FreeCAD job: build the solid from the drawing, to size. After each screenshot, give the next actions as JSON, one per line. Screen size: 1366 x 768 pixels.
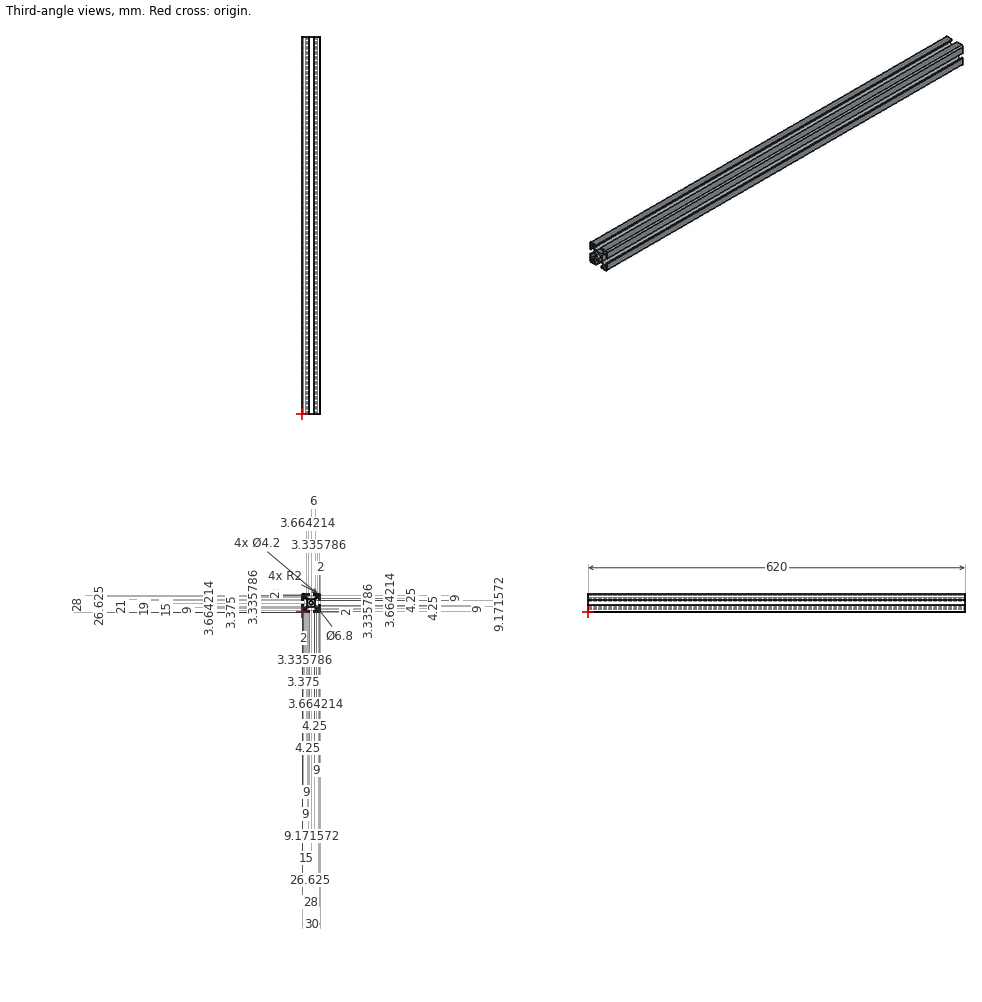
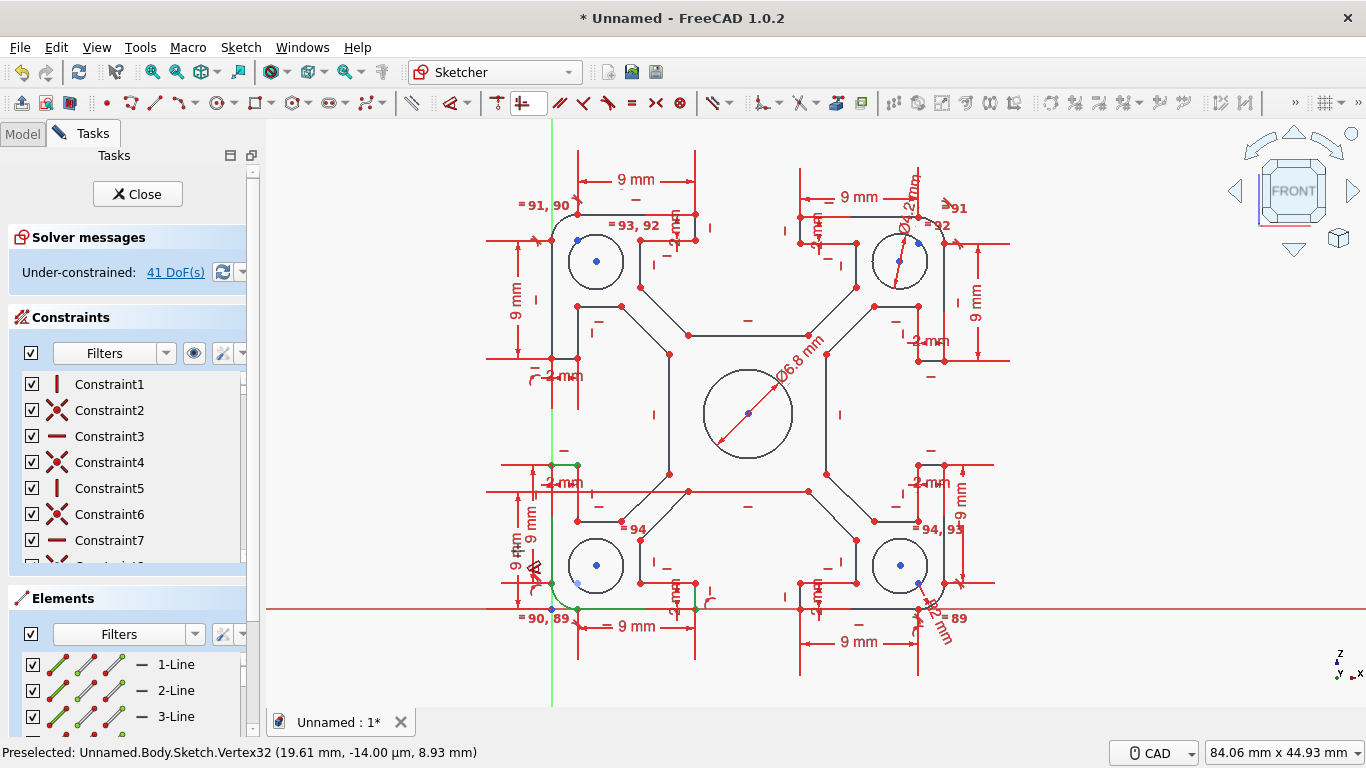
{"action": "left_click", "coordinate": [669, 475]}
{"action": "left_click", "coordinate": [610, 441]}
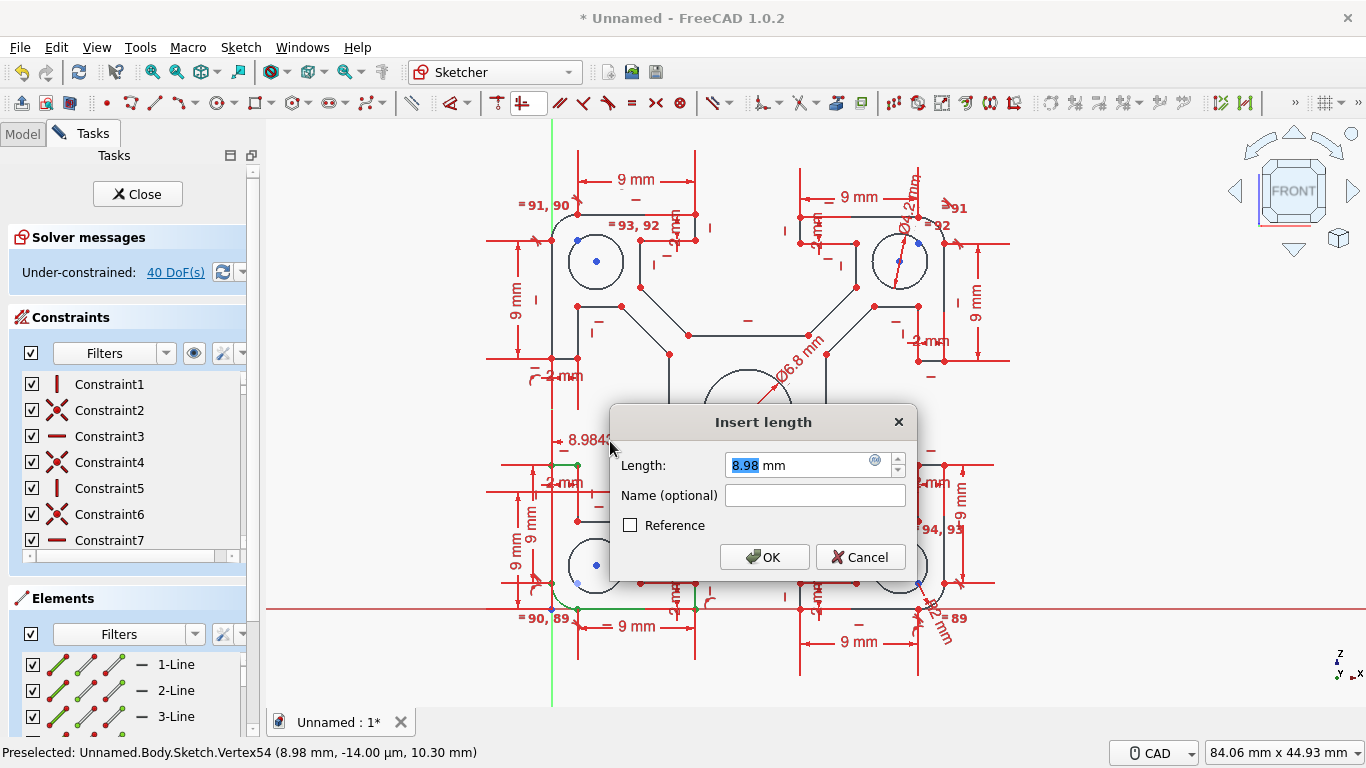
{"action": "type", "text": "9"}
{"action": "key", "text": "Return"}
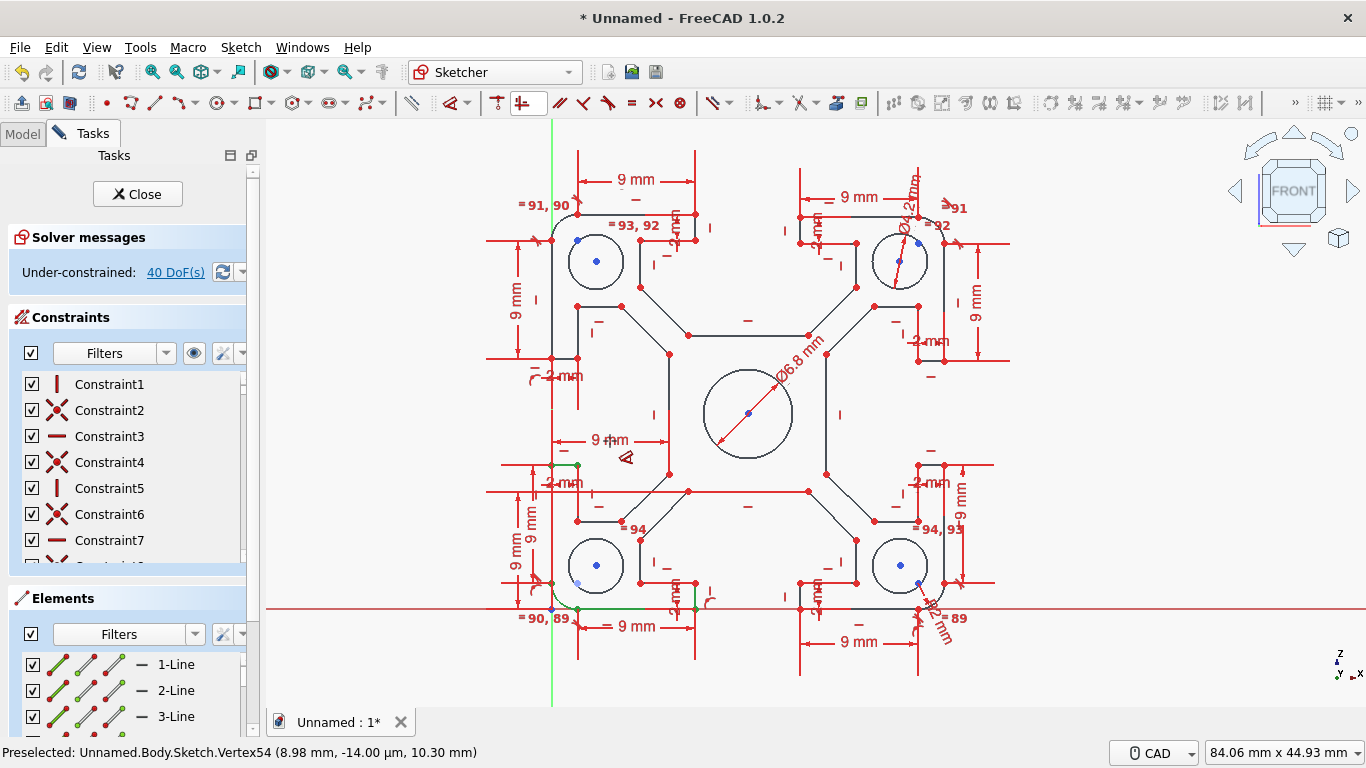
{"action": "left_click", "coordinate": [748, 414]}
{"action": "left_click", "coordinate": [719, 643]}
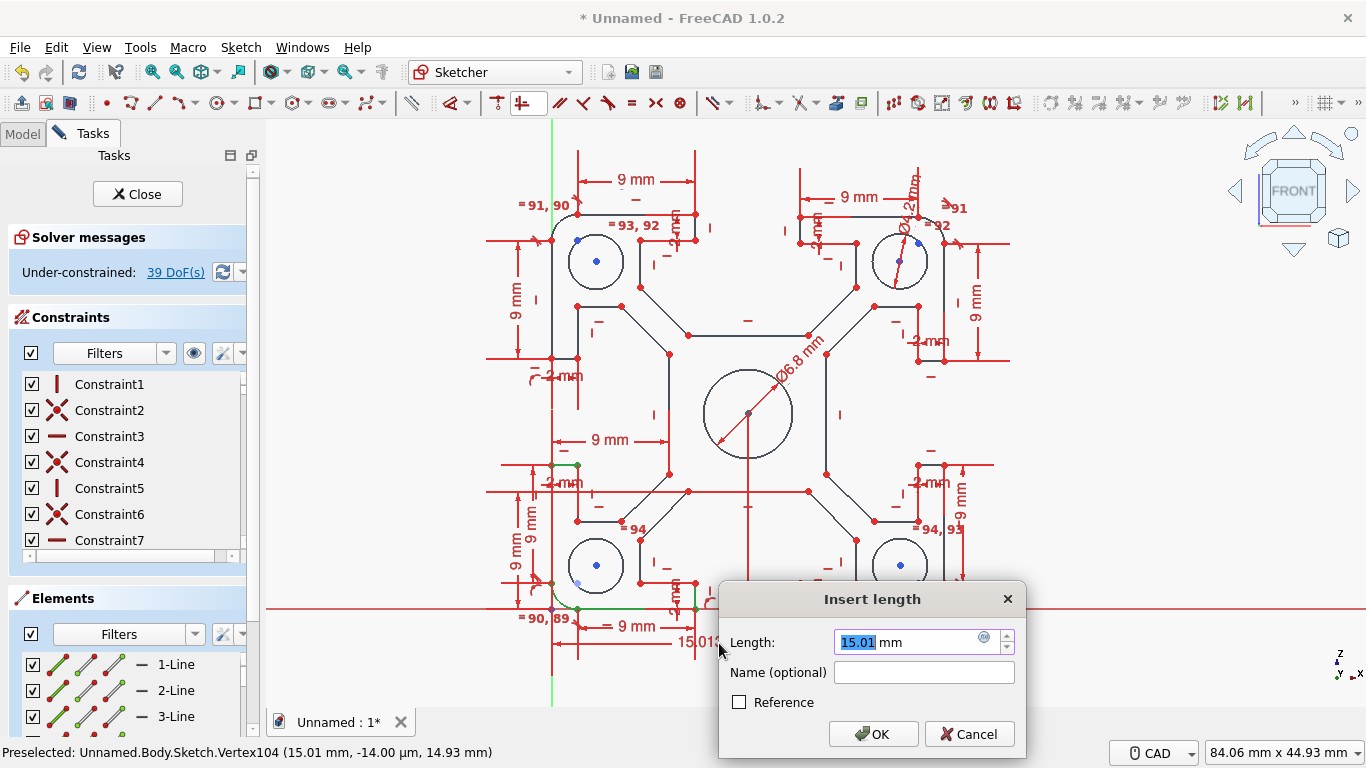
{"action": "type", "text": "15"}
{"action": "key", "text": "Return"}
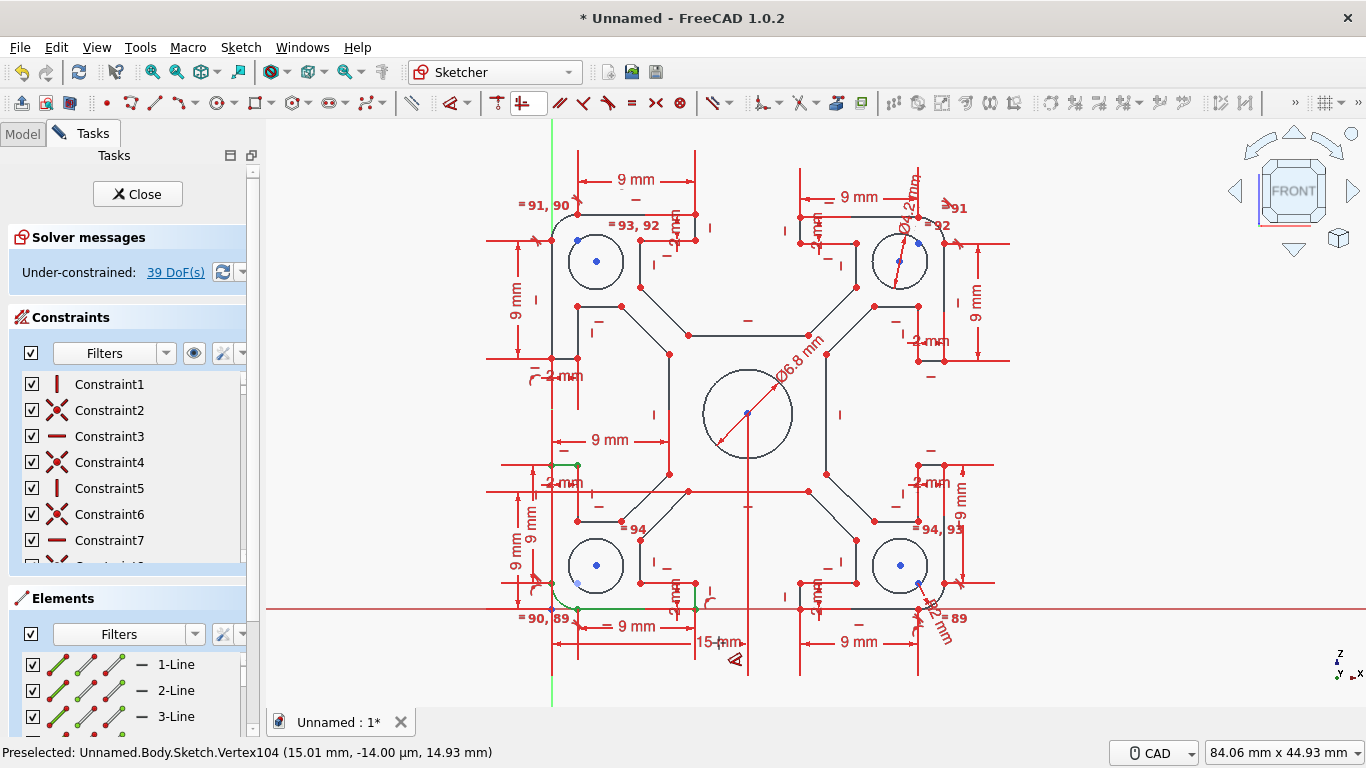
{"action": "left_click", "coordinate": [748, 414]}
{"action": "left_click", "coordinate": [518, 443]}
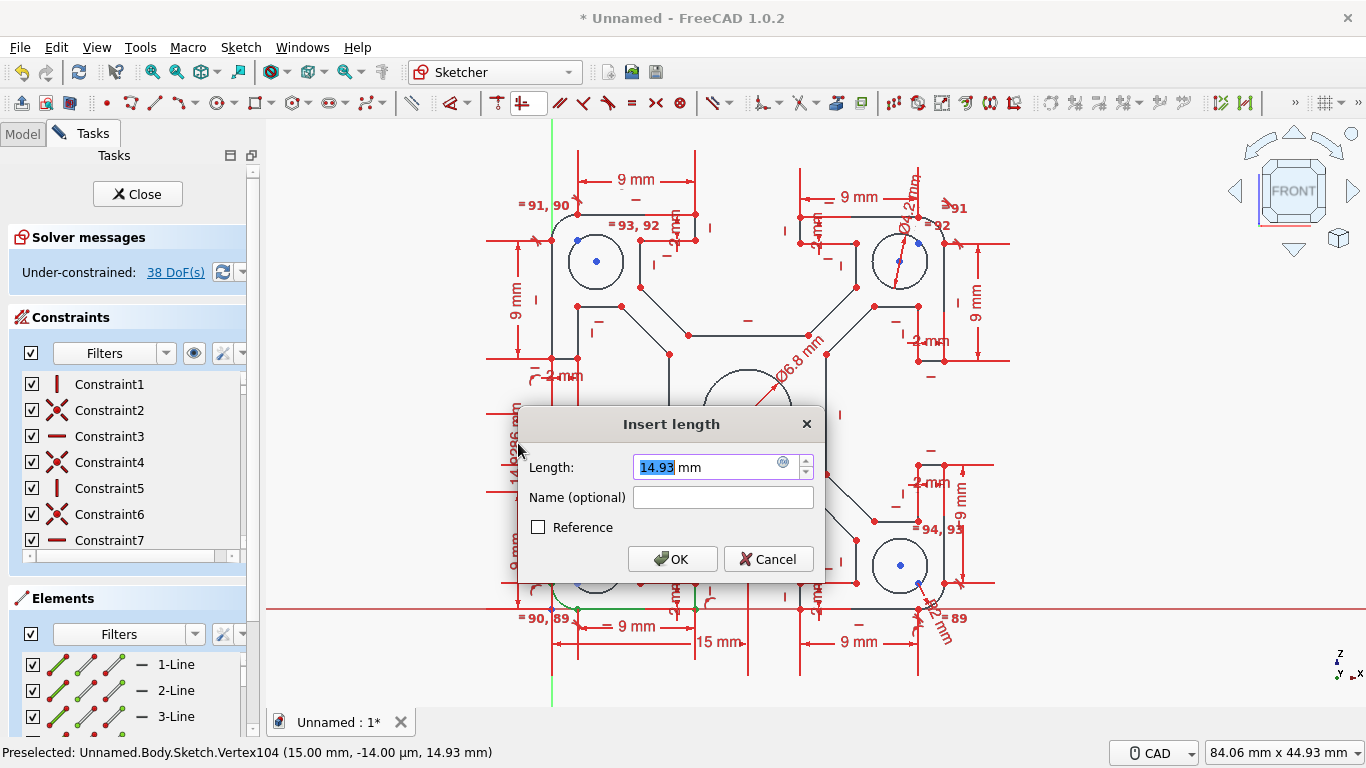
{"action": "type", "text": "15"}
{"action": "key", "text": "Return"}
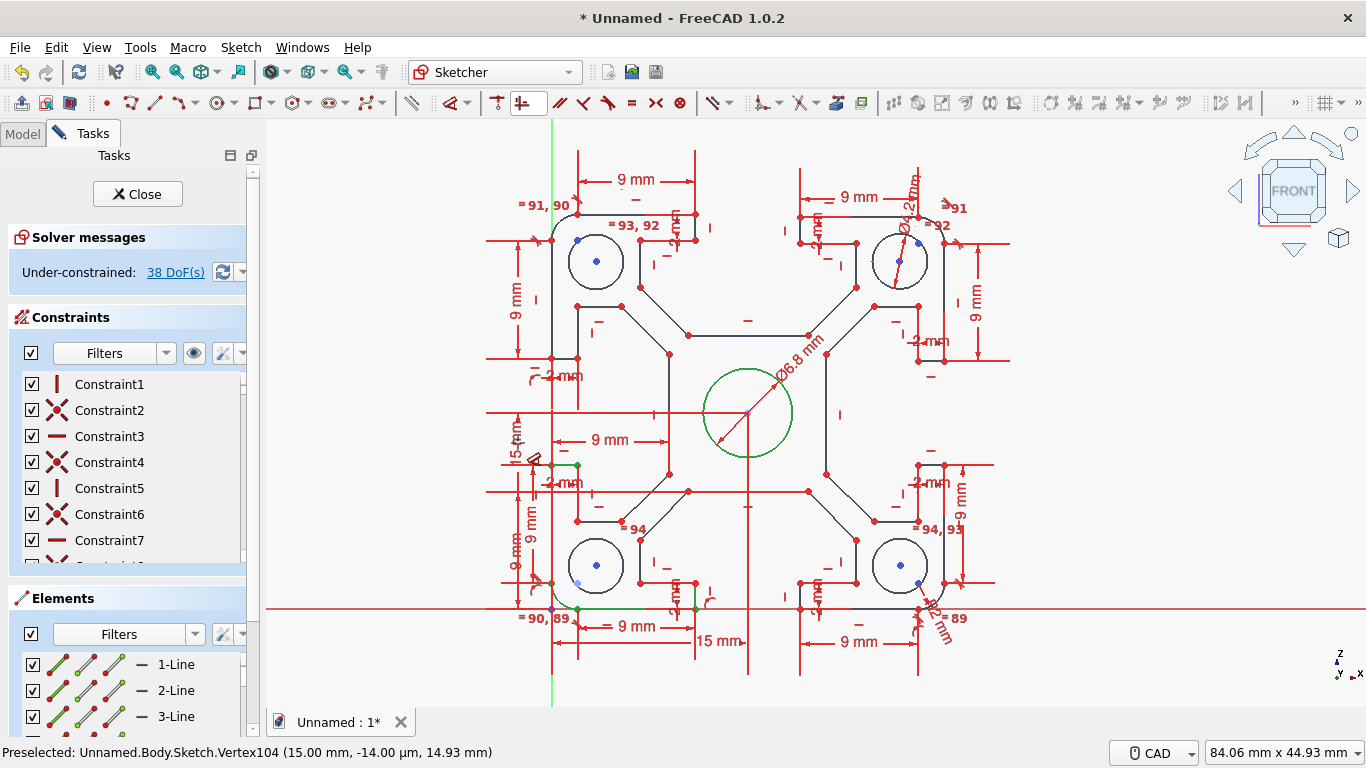
{"action": "left_click", "coordinate": [826, 355]}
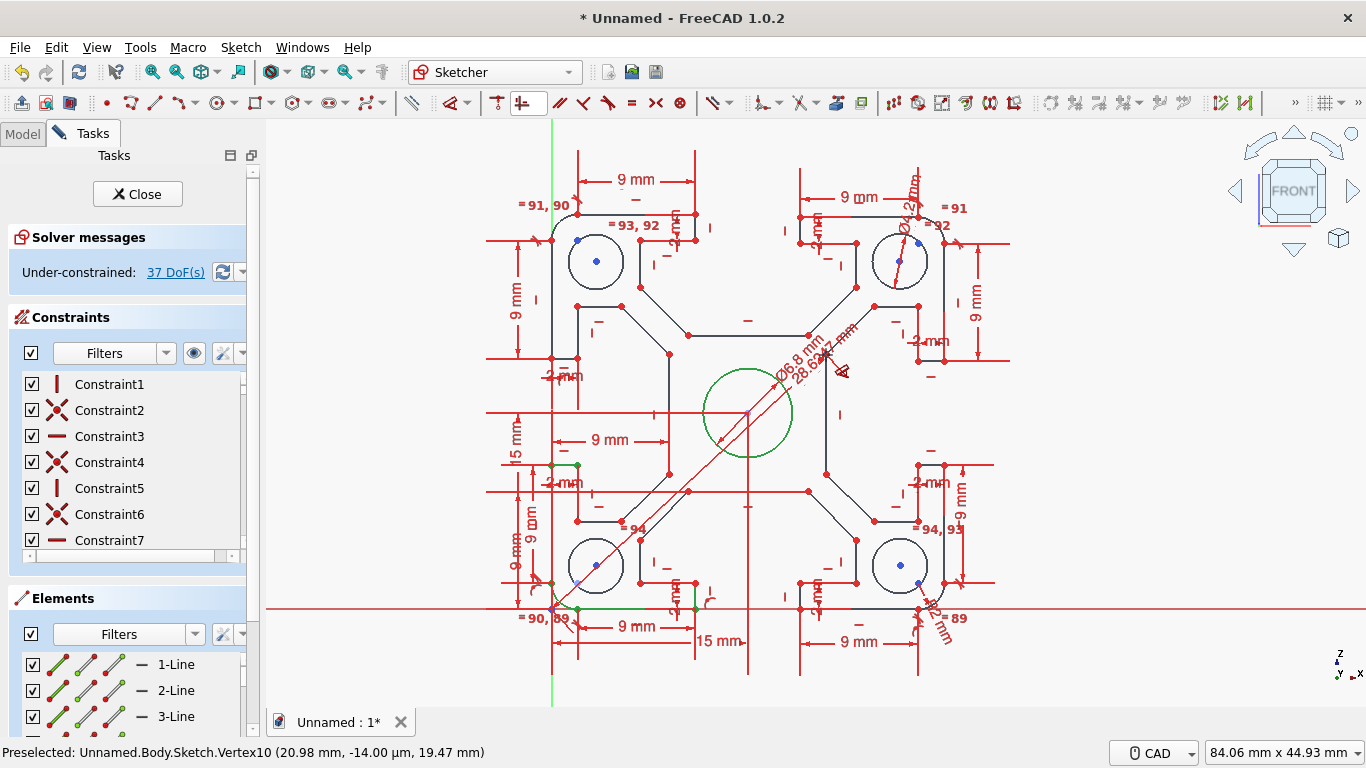
{"action": "left_click", "coordinate": [748, 413]}
{"action": "left_click", "coordinate": [787, 321]}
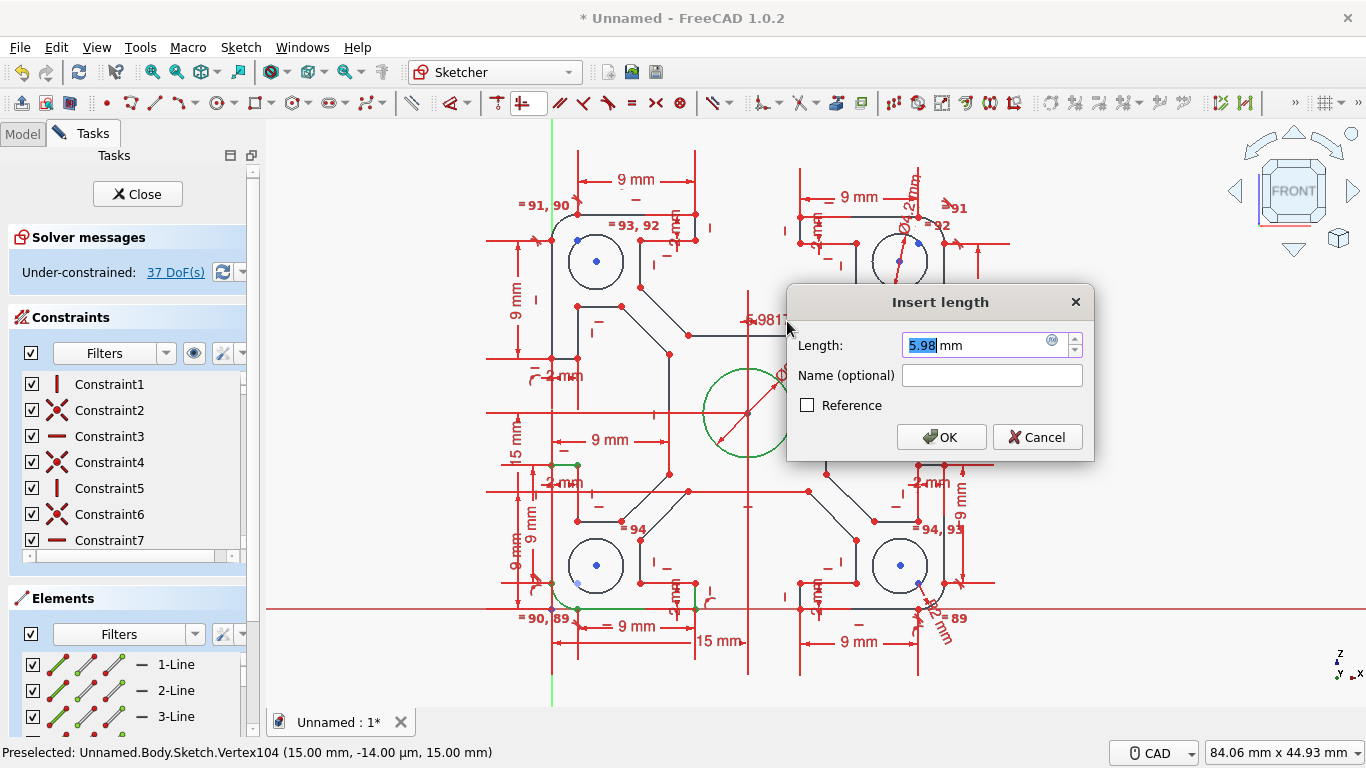
{"action": "type", "text": "6"}
{"action": "key", "text": "Return"}